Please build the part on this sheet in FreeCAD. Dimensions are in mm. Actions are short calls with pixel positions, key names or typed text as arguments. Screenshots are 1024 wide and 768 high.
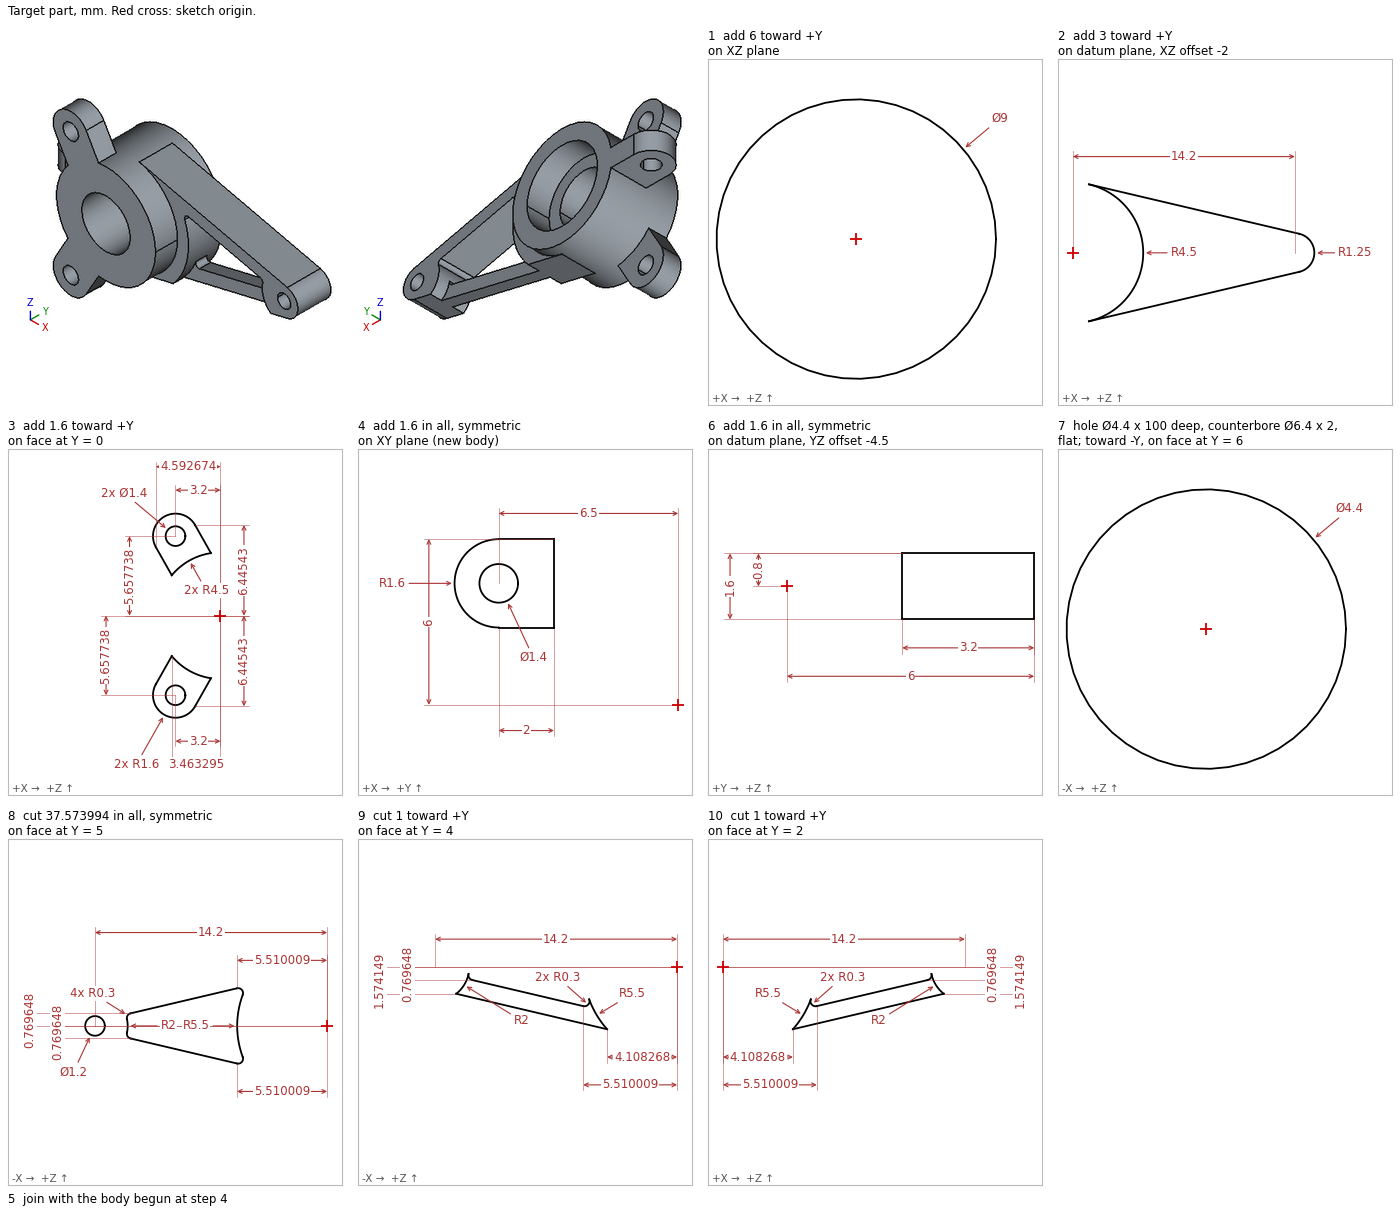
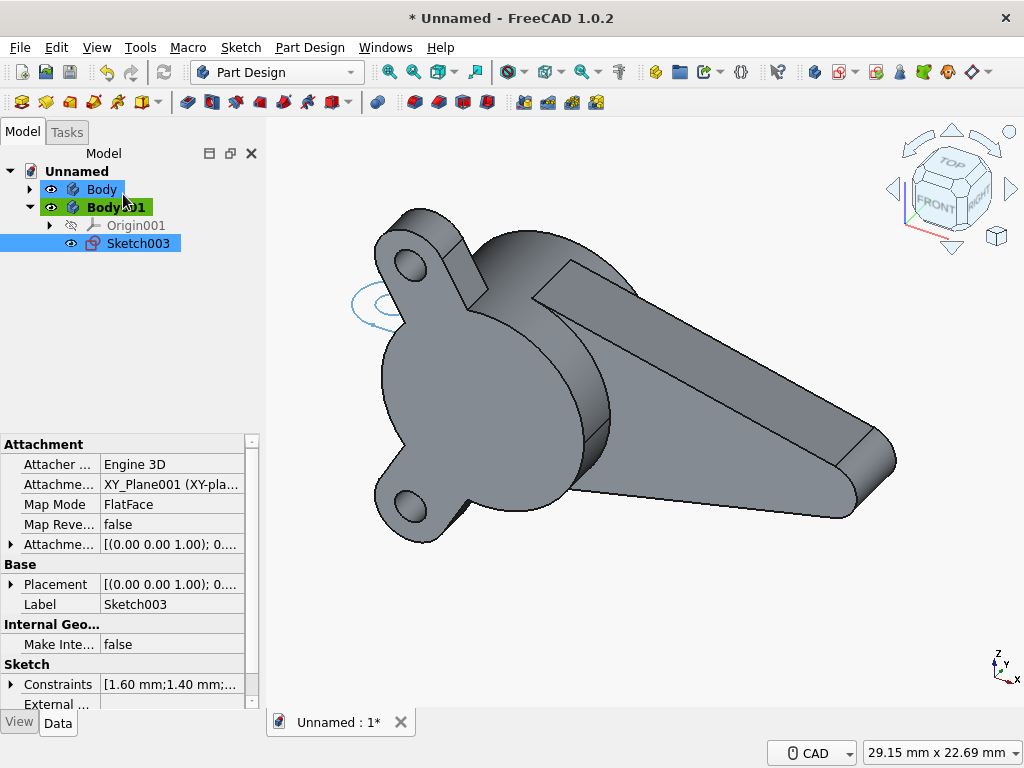
click(22, 102)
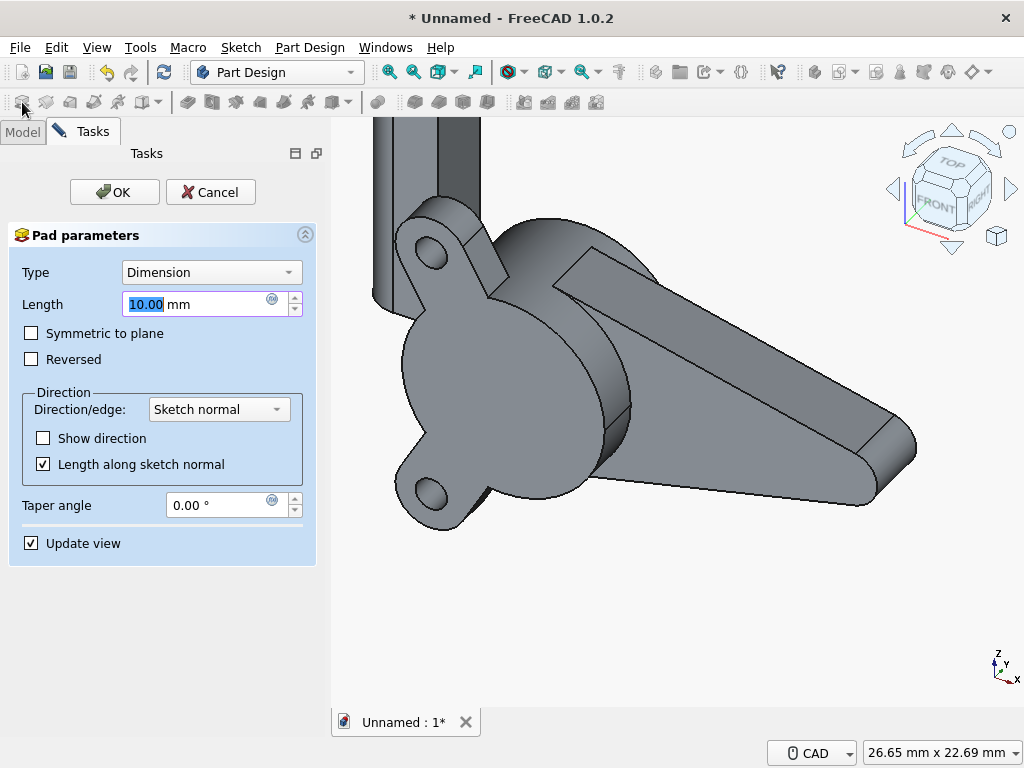
text(1.6)
key(Tab)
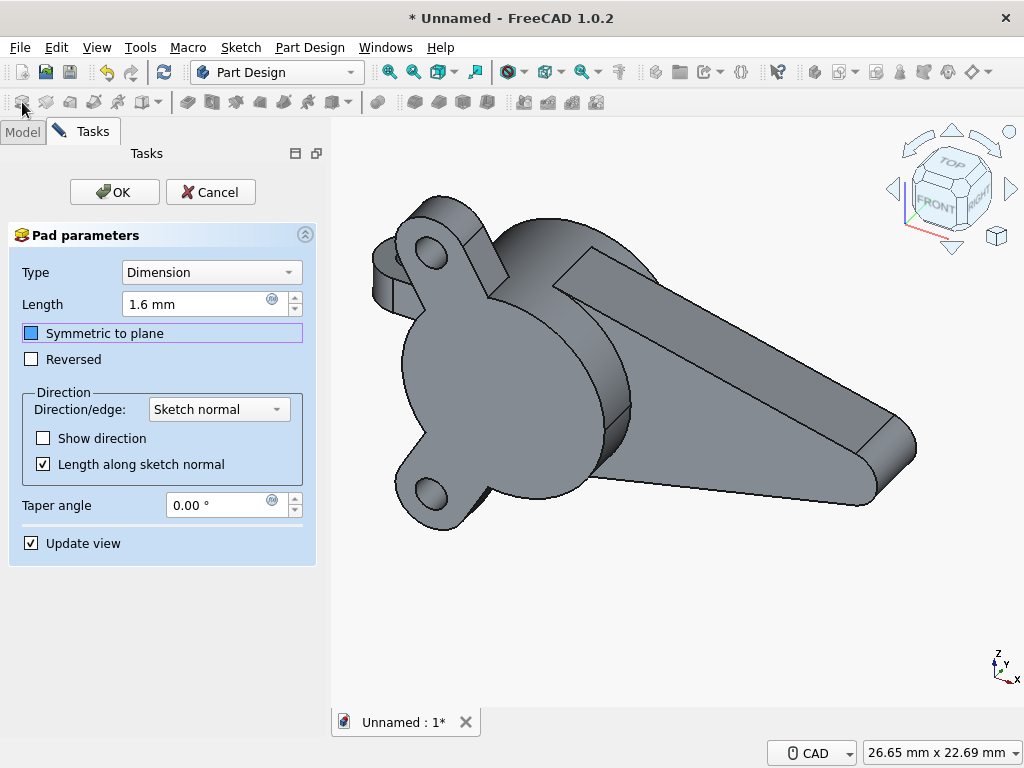
click(30, 333)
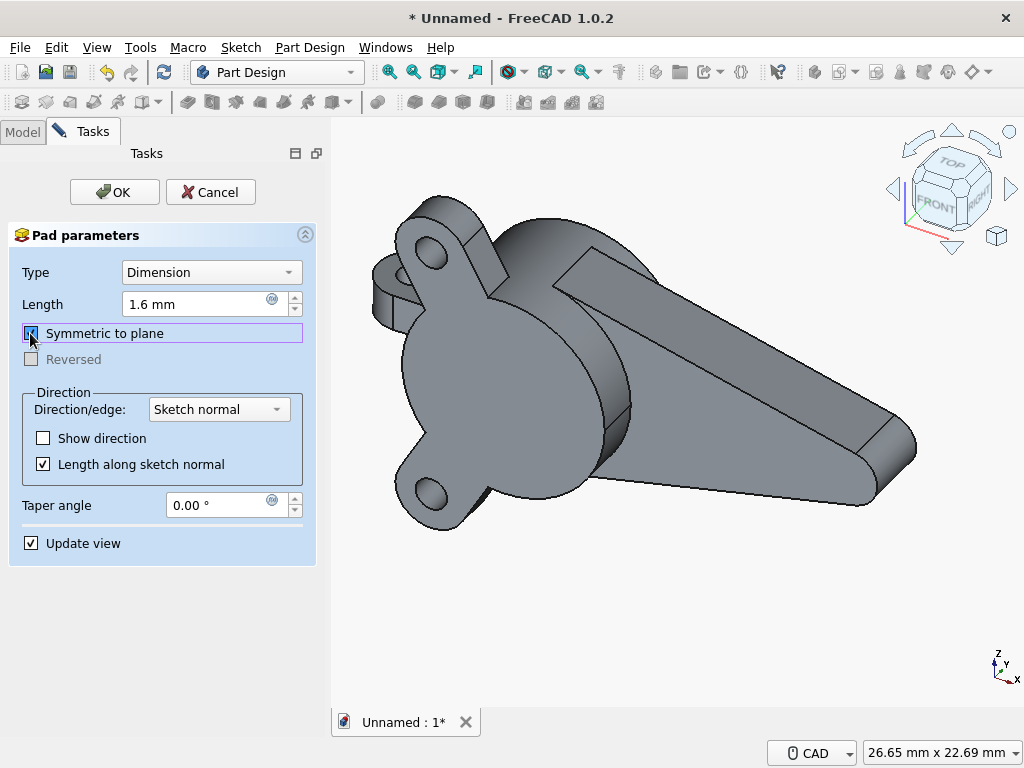
click(115, 192)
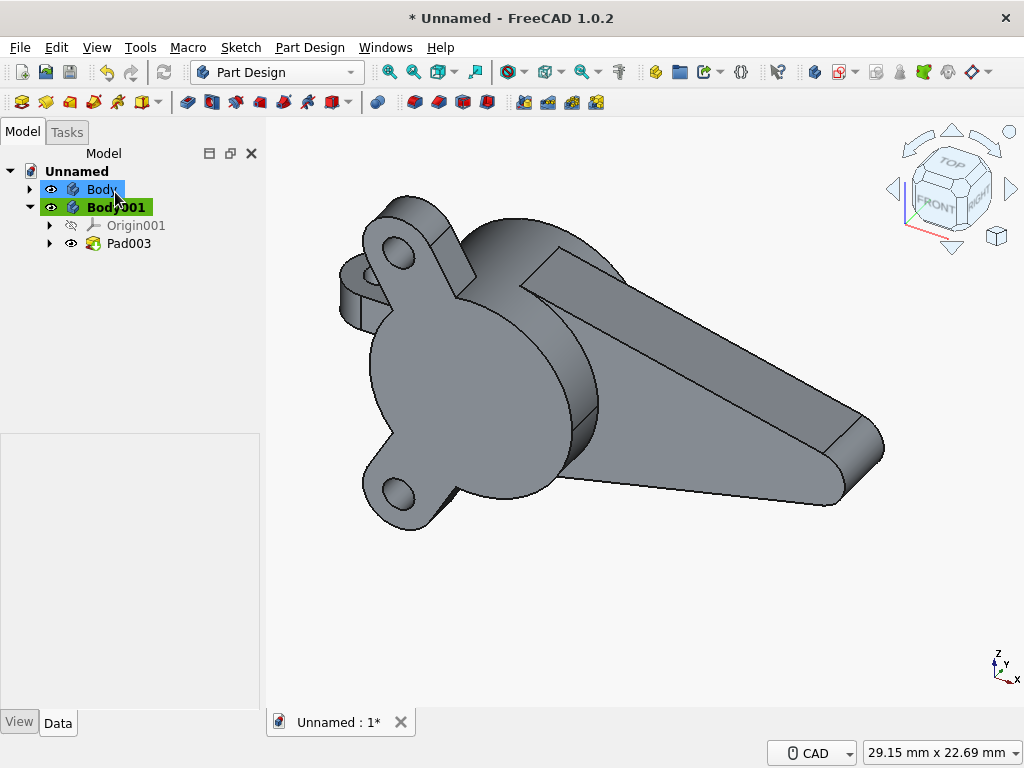
key(v)
key(f)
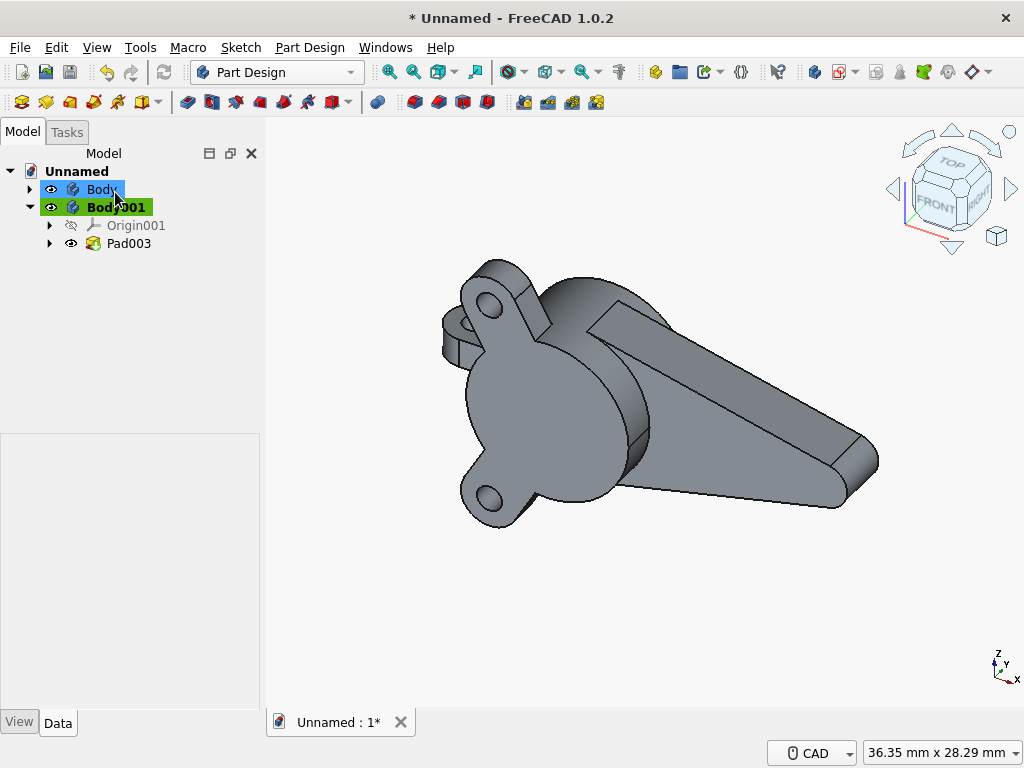
double_click(96, 189)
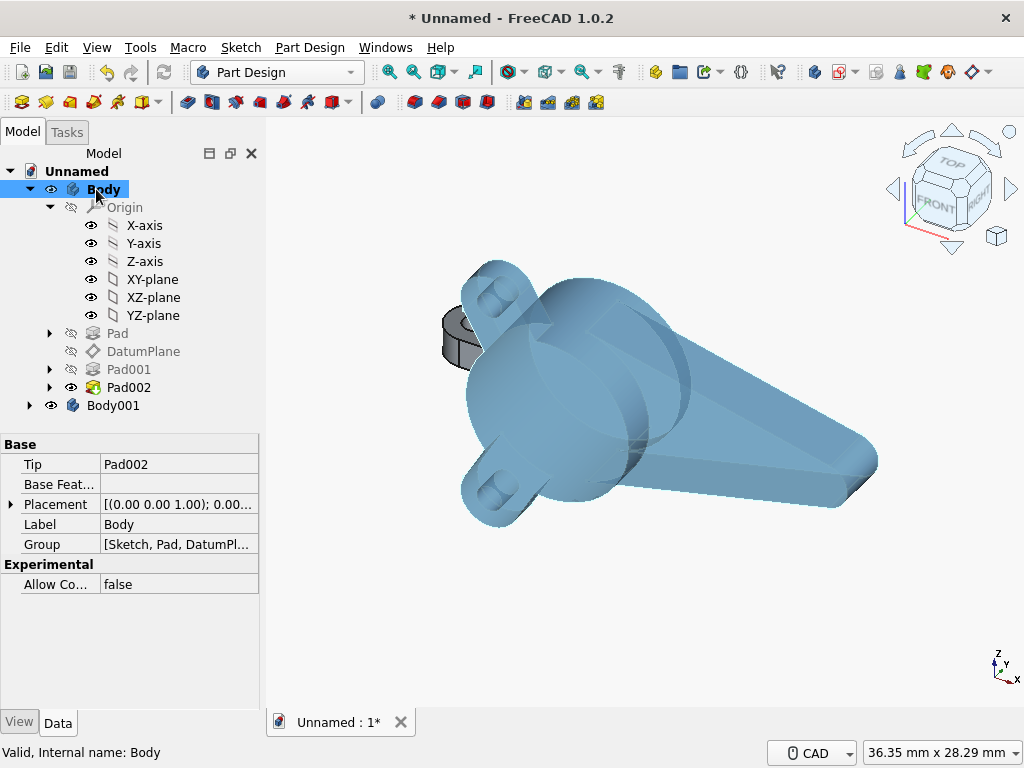
click(96, 189)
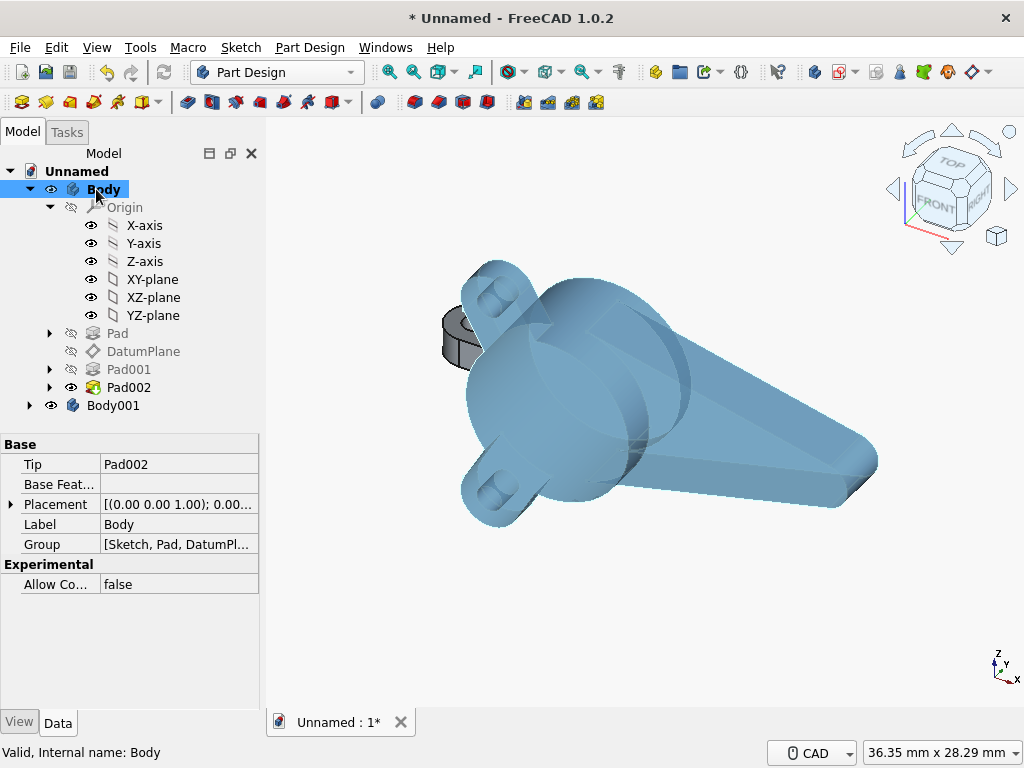
click(146, 584)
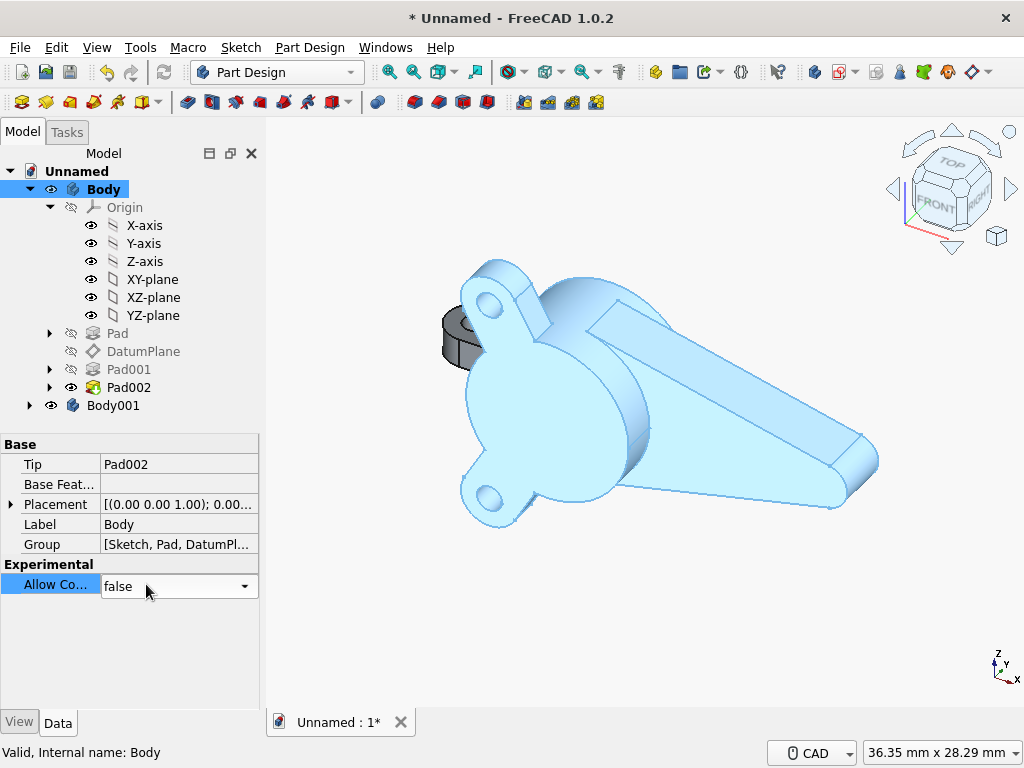
click(146, 584)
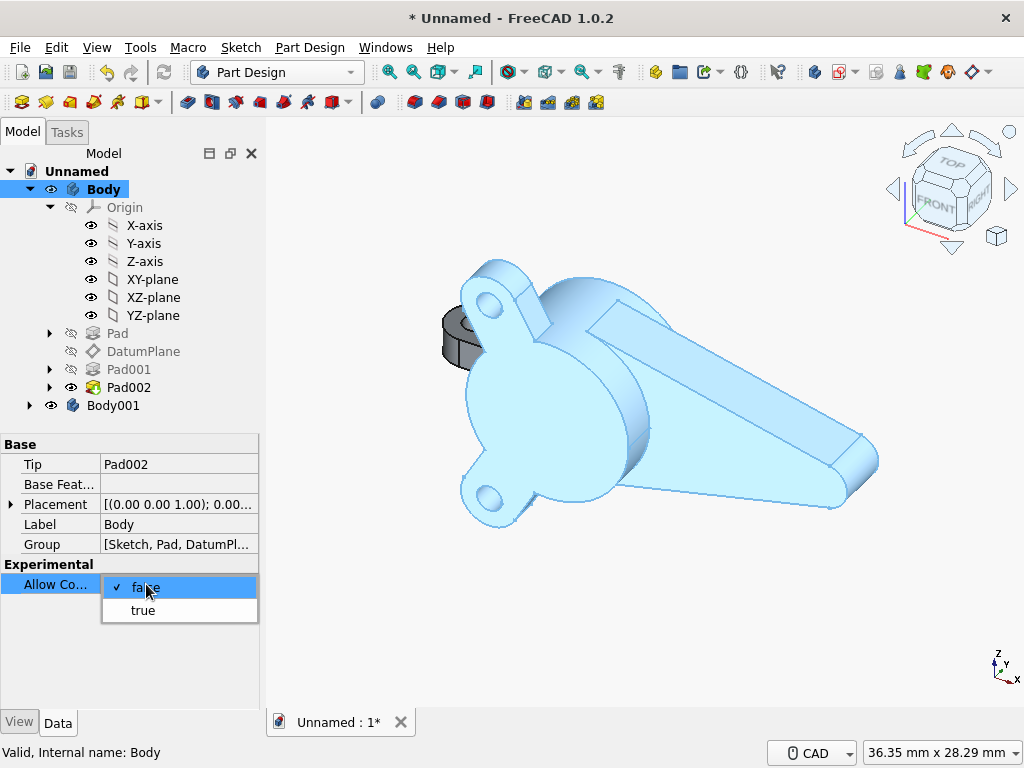
click(179, 610)
key(Return)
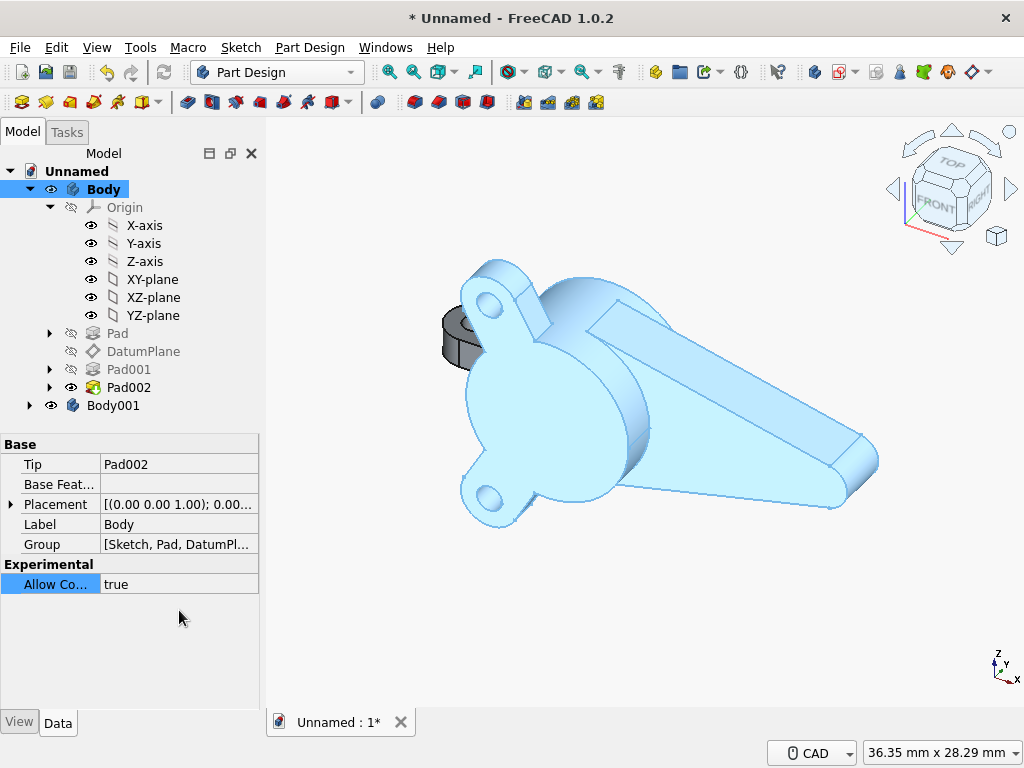
click(96, 405)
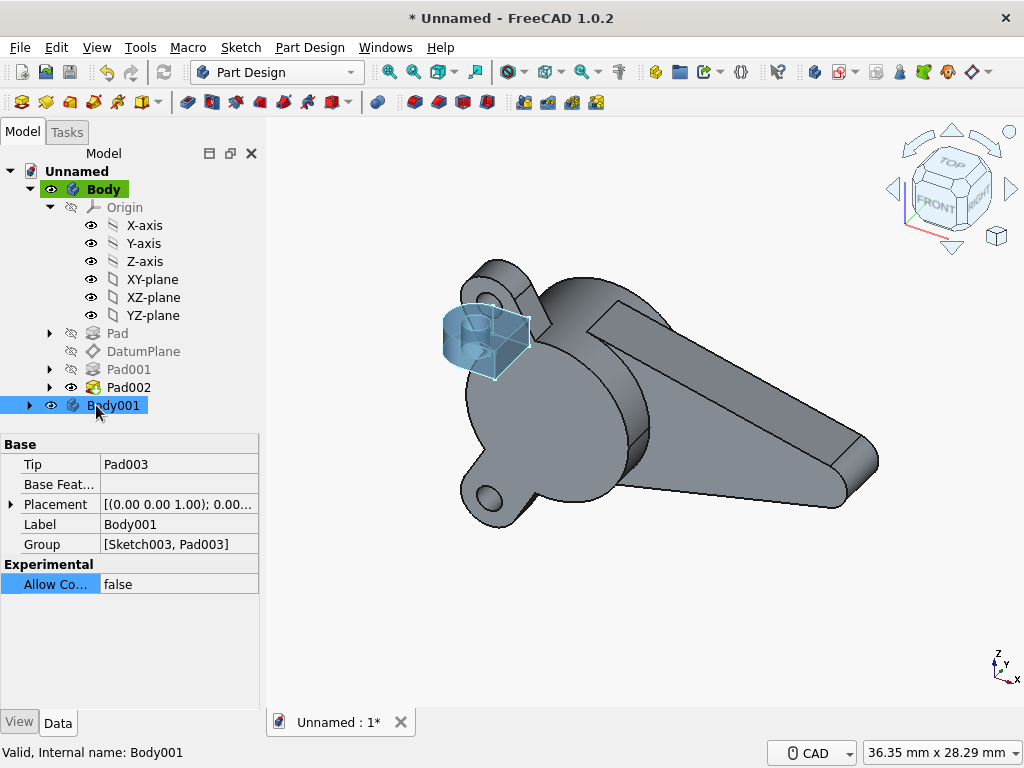
click(378, 102)